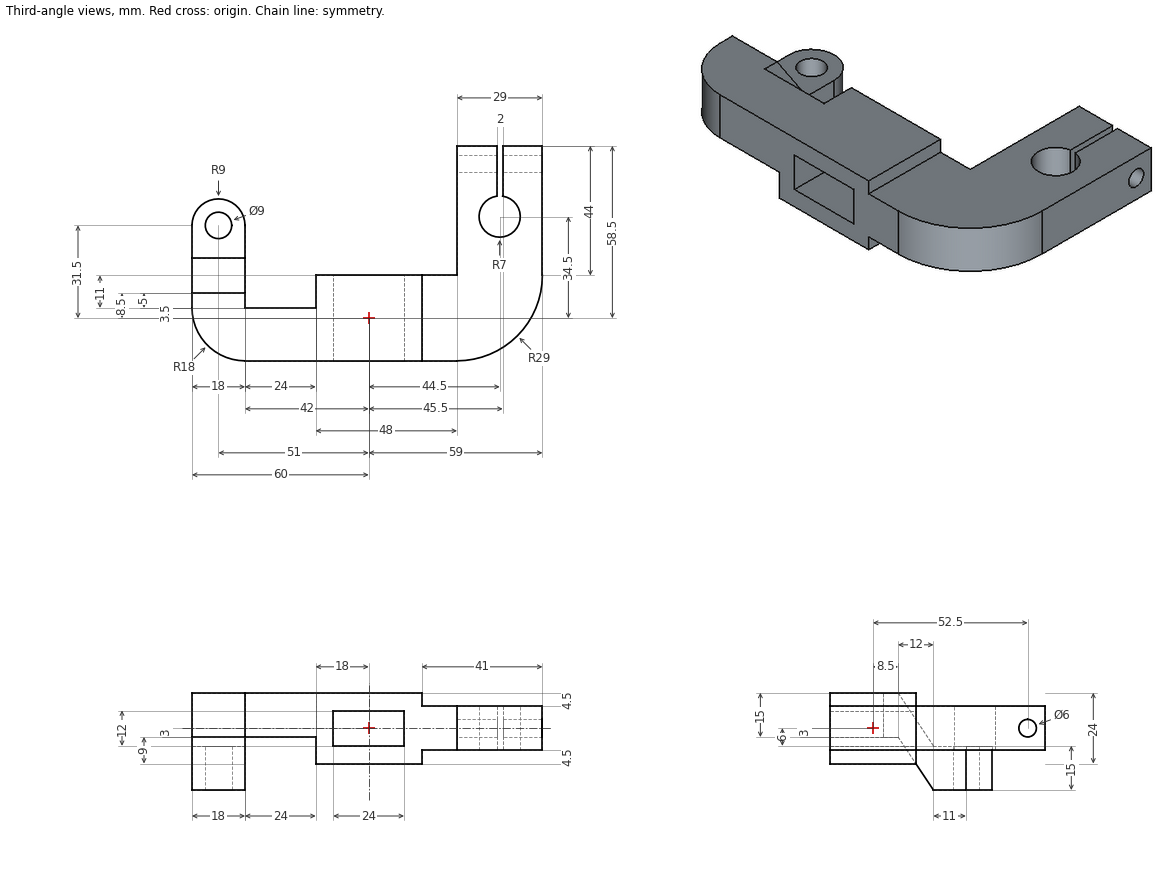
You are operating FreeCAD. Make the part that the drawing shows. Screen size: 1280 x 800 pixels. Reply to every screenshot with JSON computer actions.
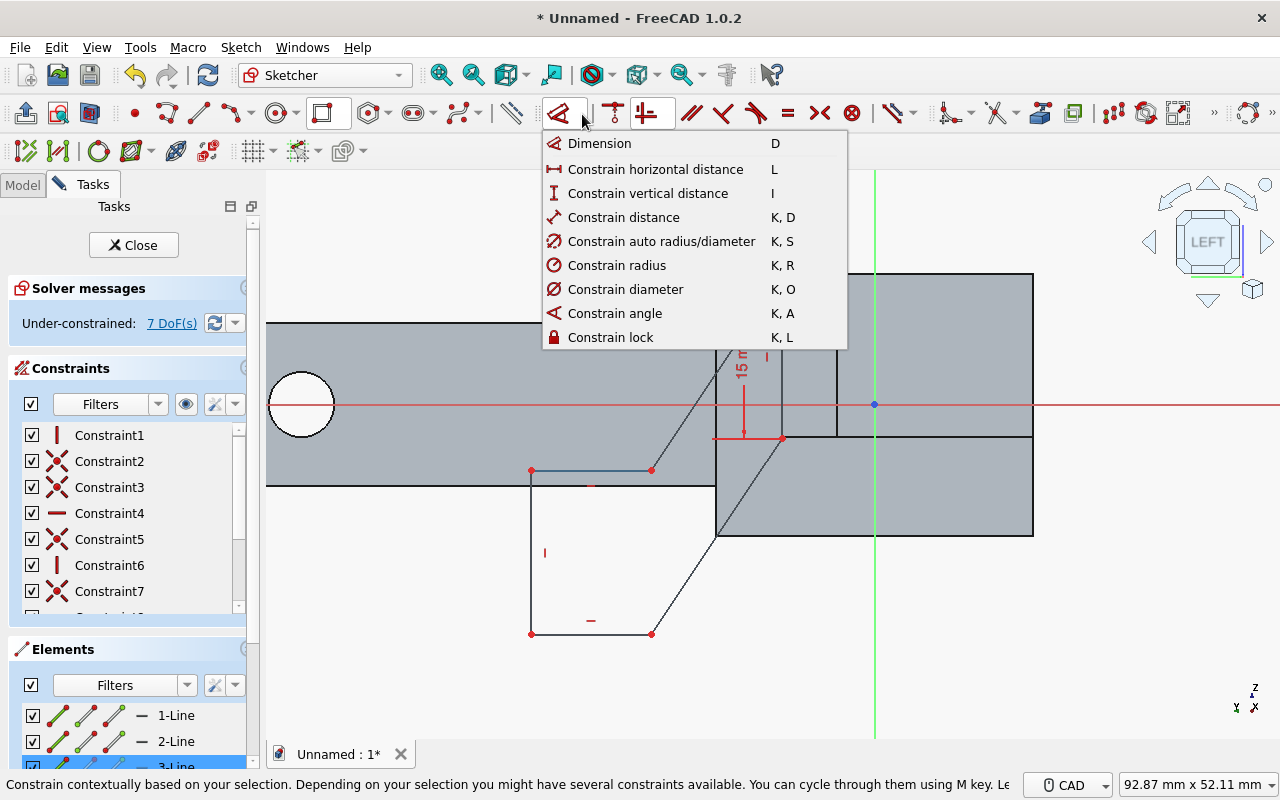
{"action": "left_click", "coordinate": [695, 169]}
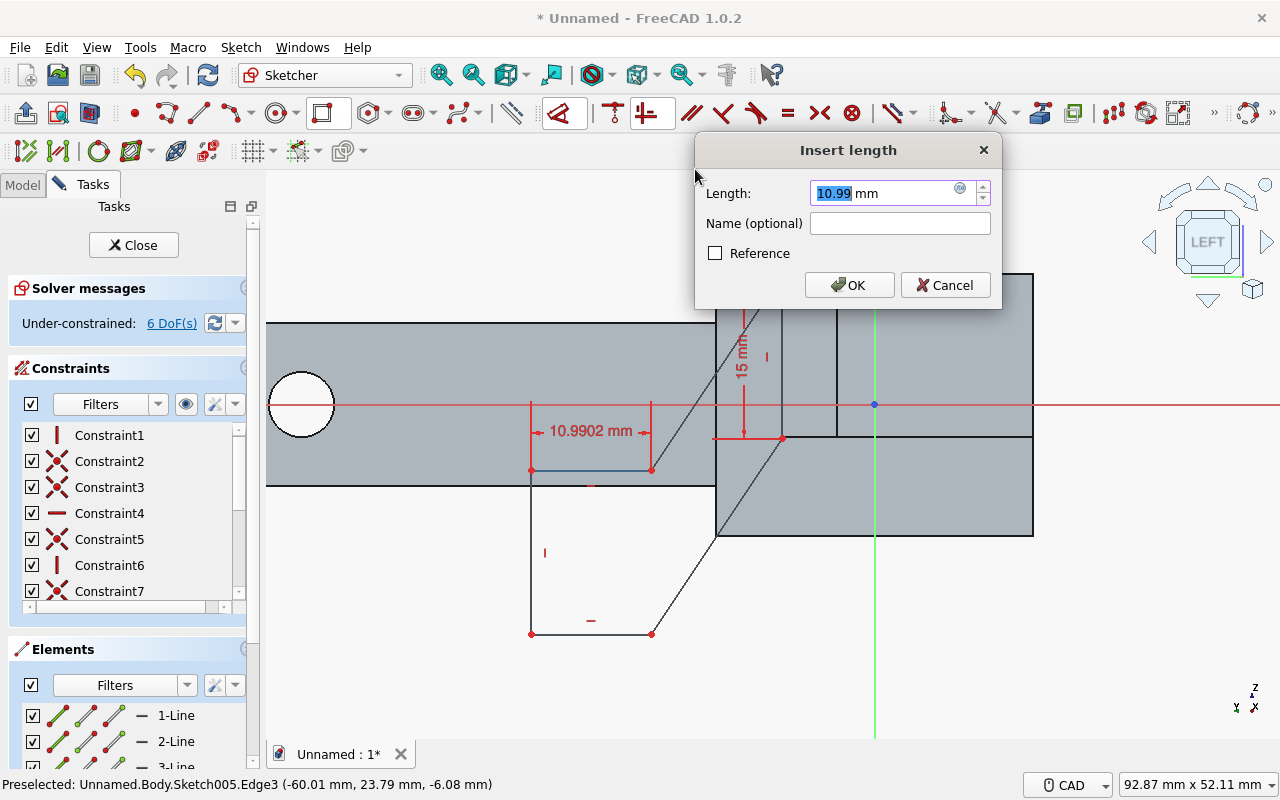
{"action": "type", "text": "11"}
{"action": "key", "text": "Return"}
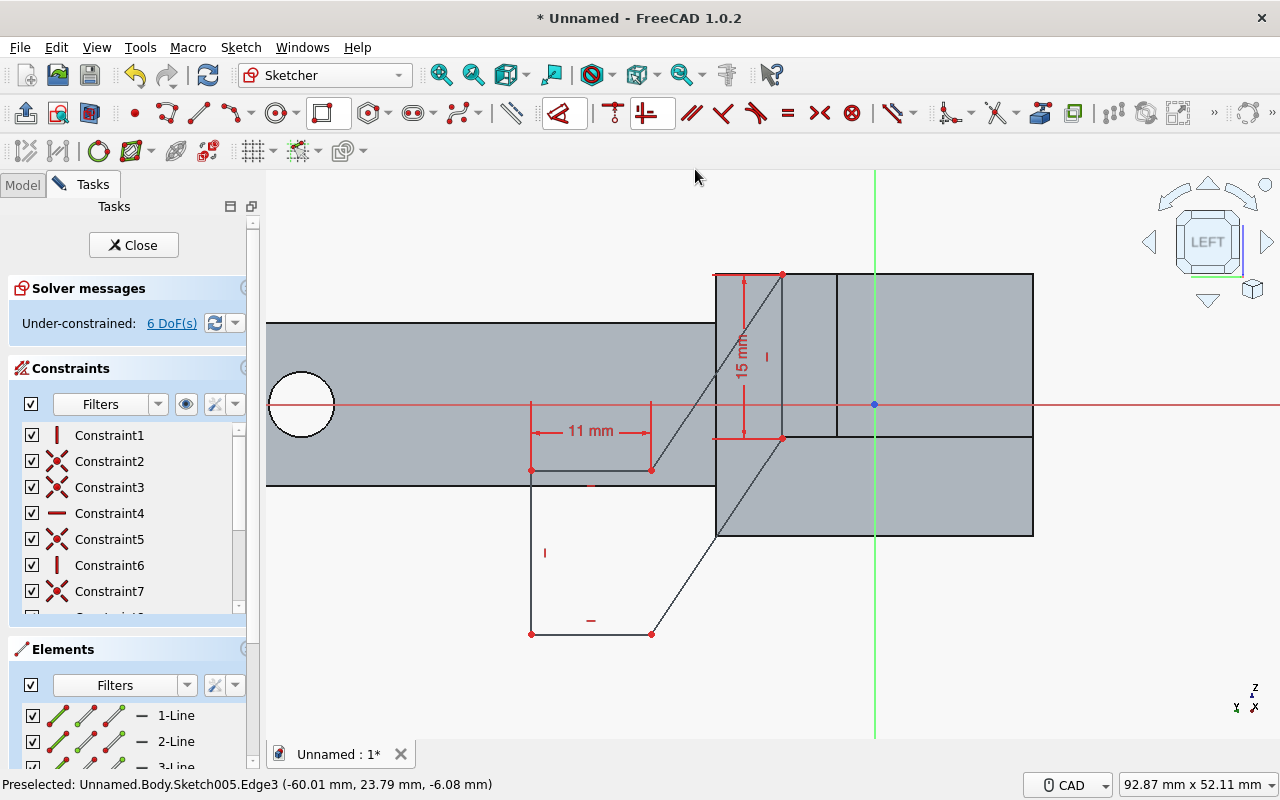
{"action": "left_click", "coordinate": [531, 520]}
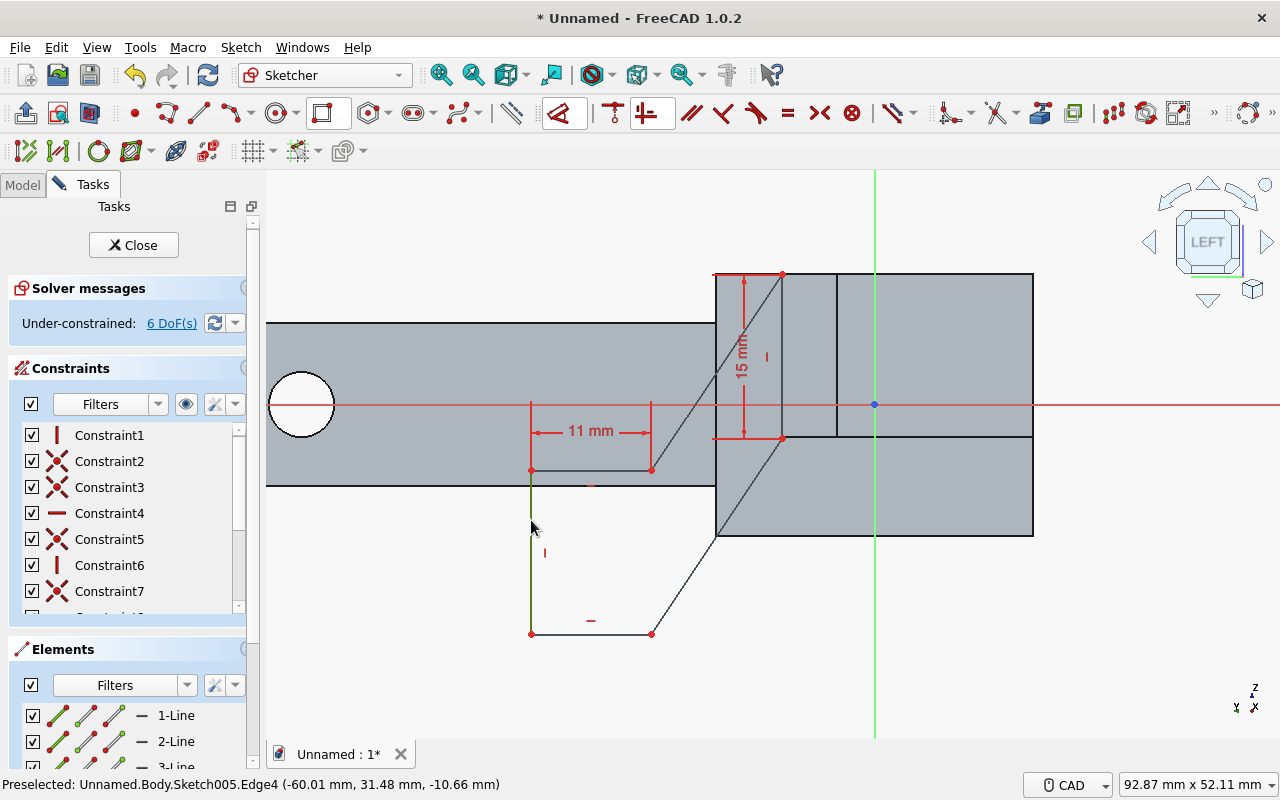
{"action": "key", "text": "i"}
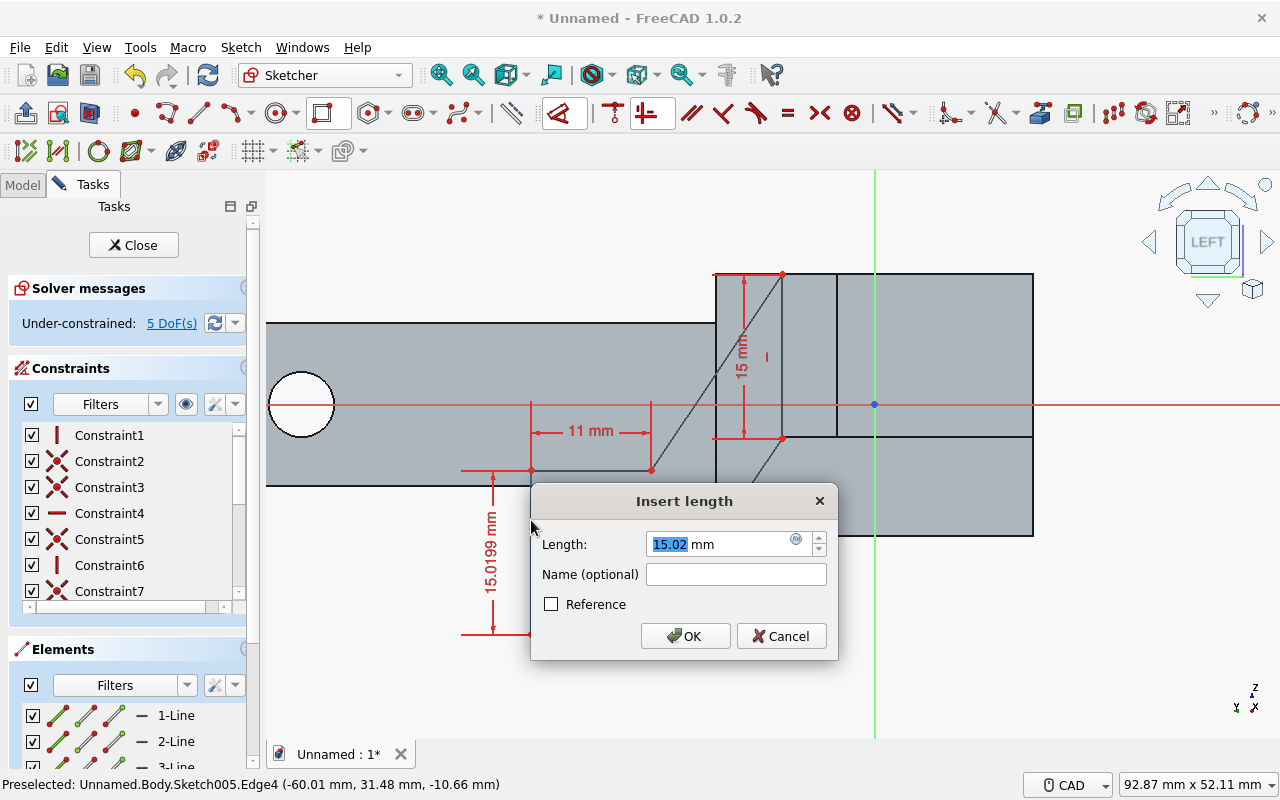
{"action": "type", "text": "15"}
{"action": "key", "text": "Return"}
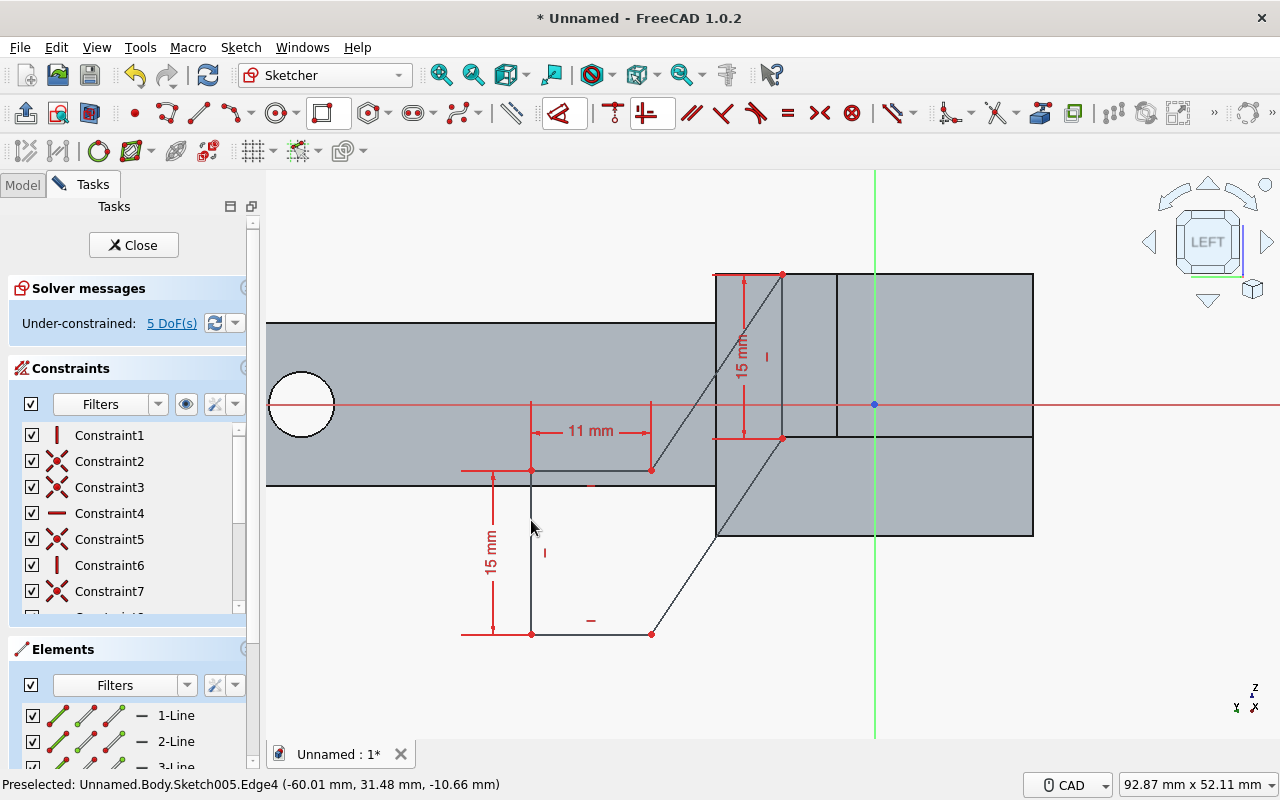
{"action": "left_click", "coordinate": [567, 635]}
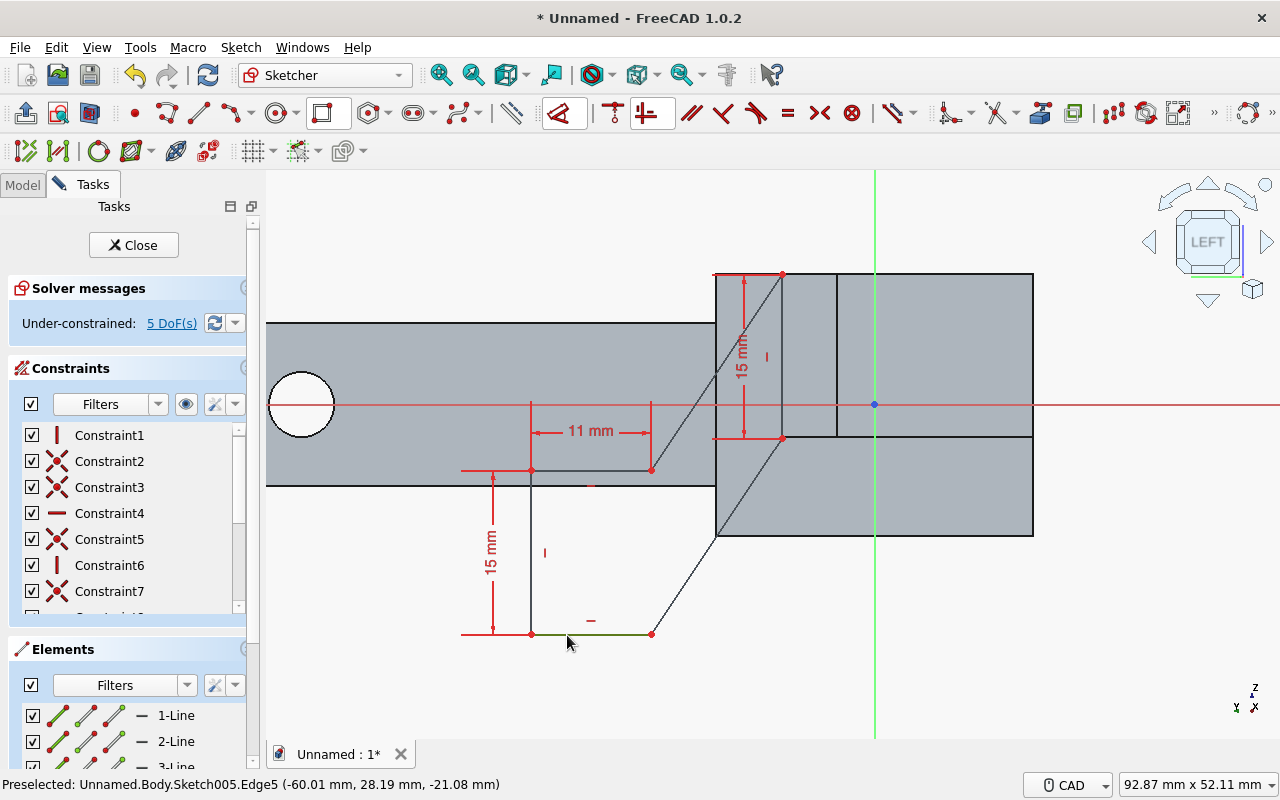
{"action": "left_click", "coordinate": [582, 114]}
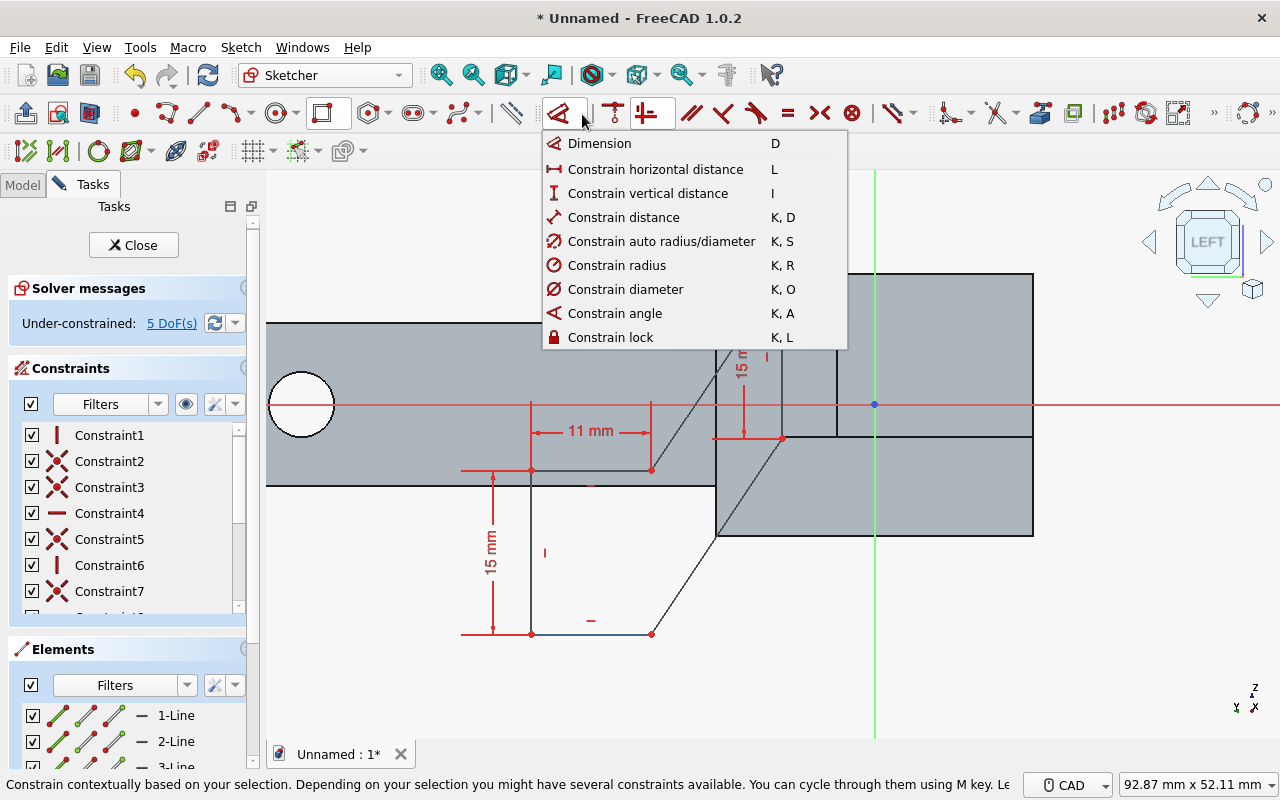
{"action": "left_click", "coordinate": [695, 169]}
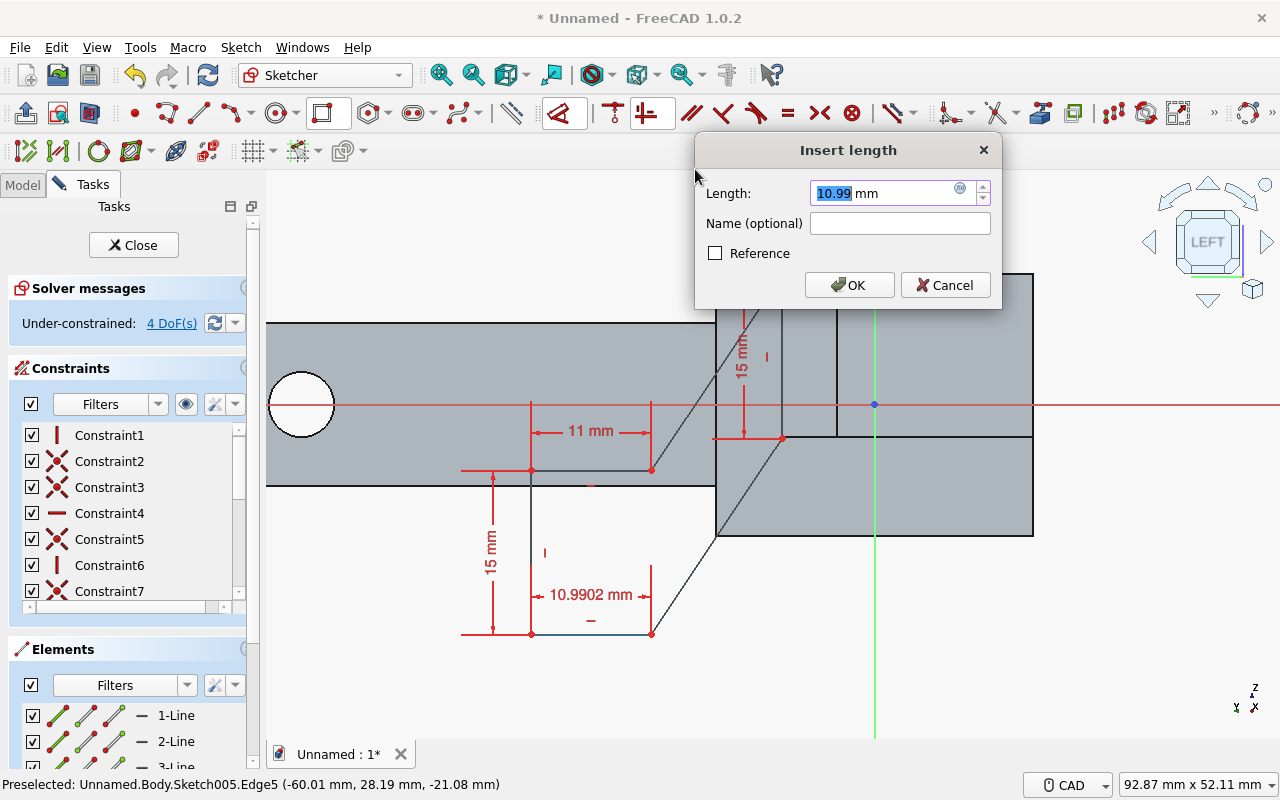
{"action": "type", "text": "11"}
{"action": "key", "text": "Return"}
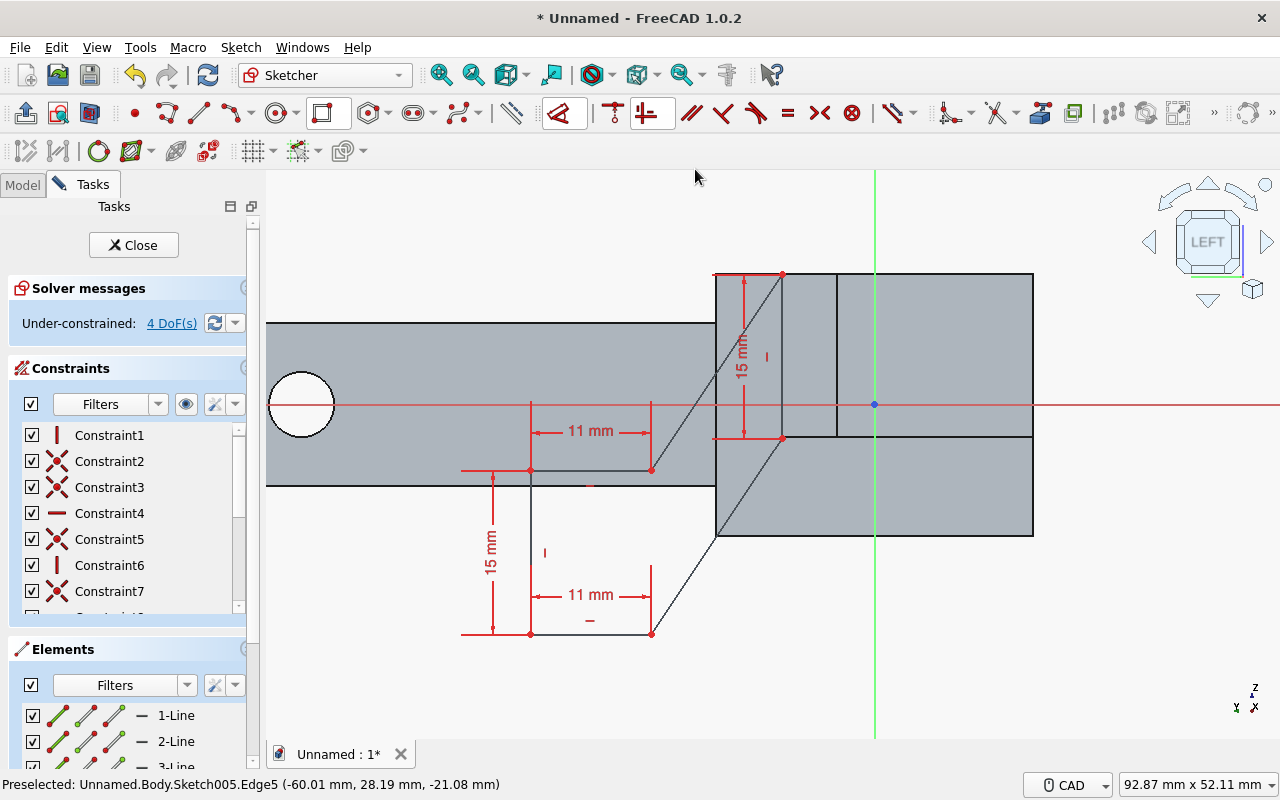
{"action": "left_click", "coordinate": [782, 439]}